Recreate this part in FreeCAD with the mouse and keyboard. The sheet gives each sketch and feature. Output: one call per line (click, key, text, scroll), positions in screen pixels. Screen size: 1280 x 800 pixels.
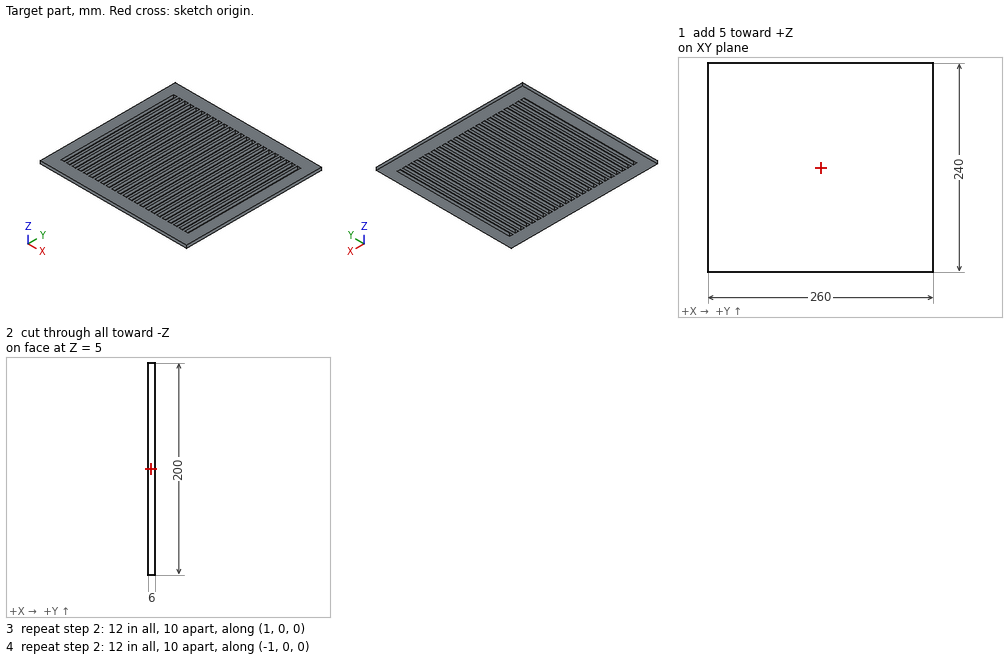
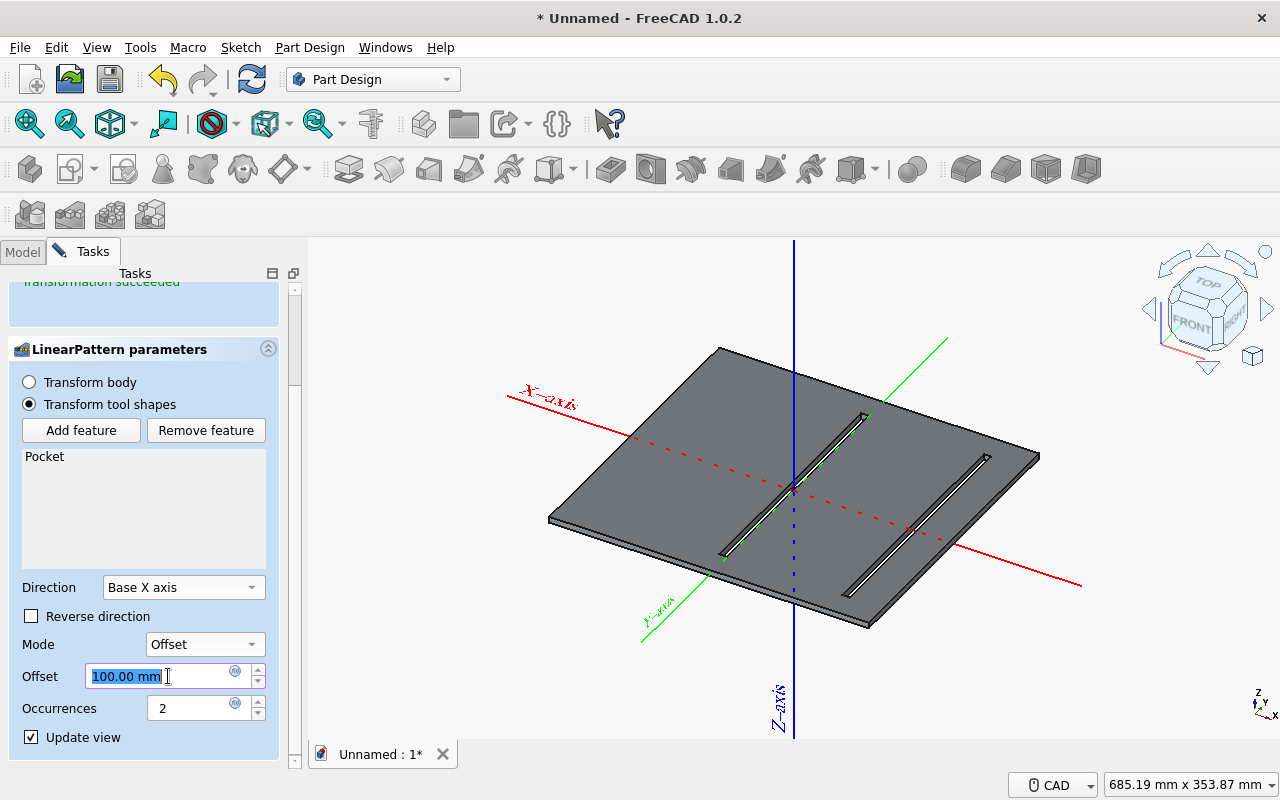
text(10)
key(Tab)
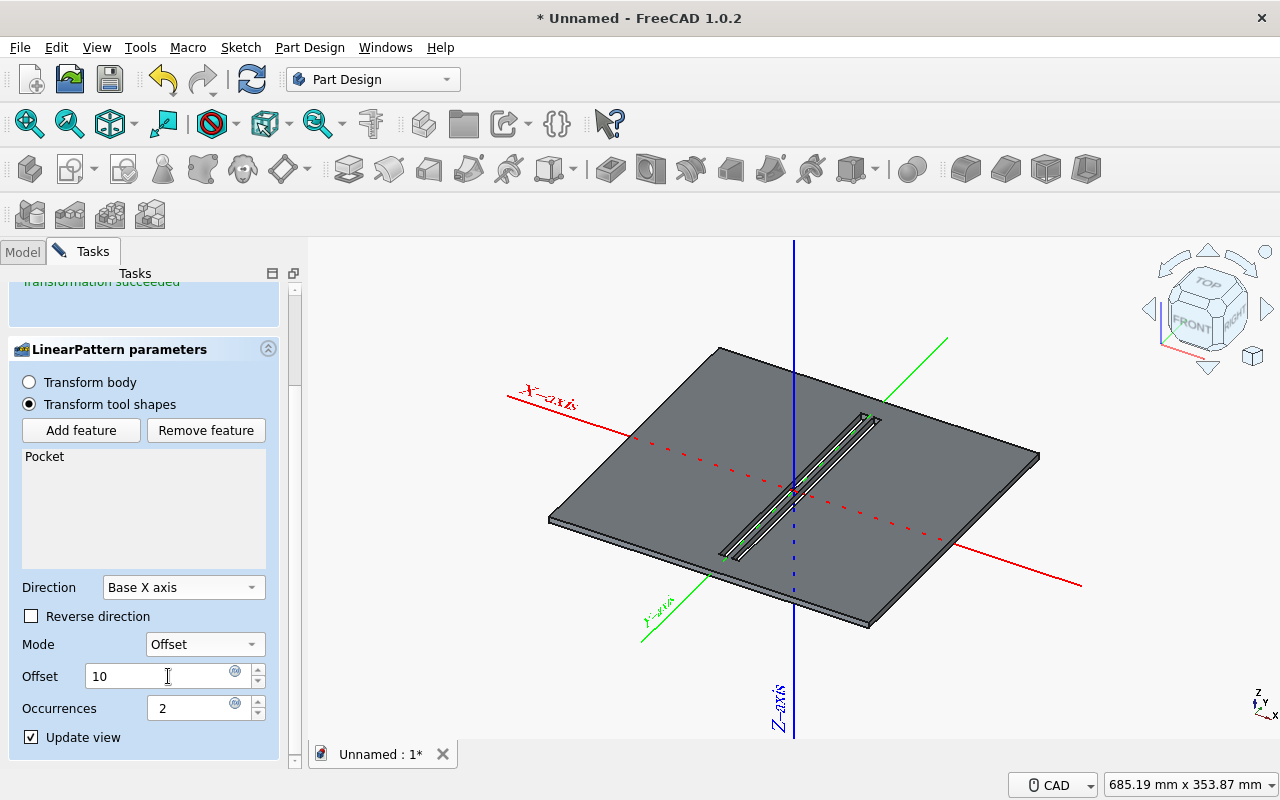
triple_click(198, 708)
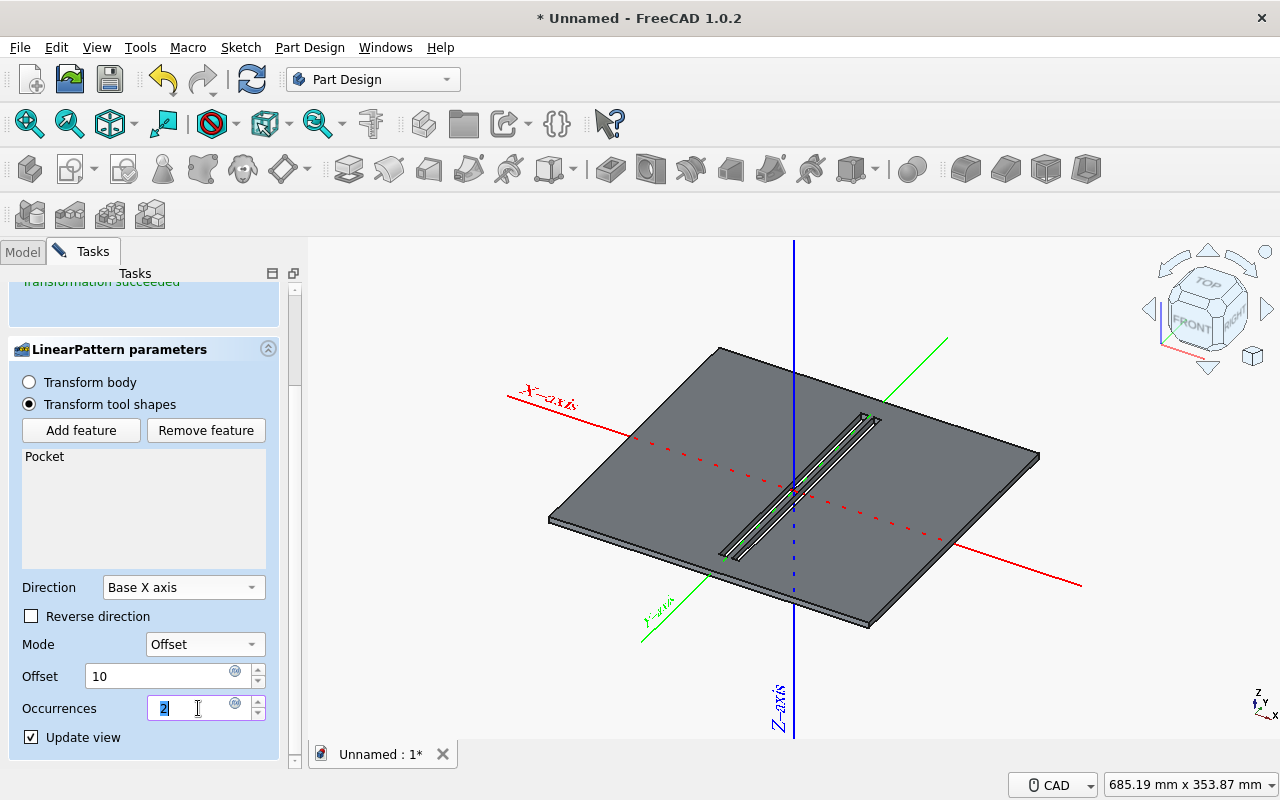
text(12)
key(Tab)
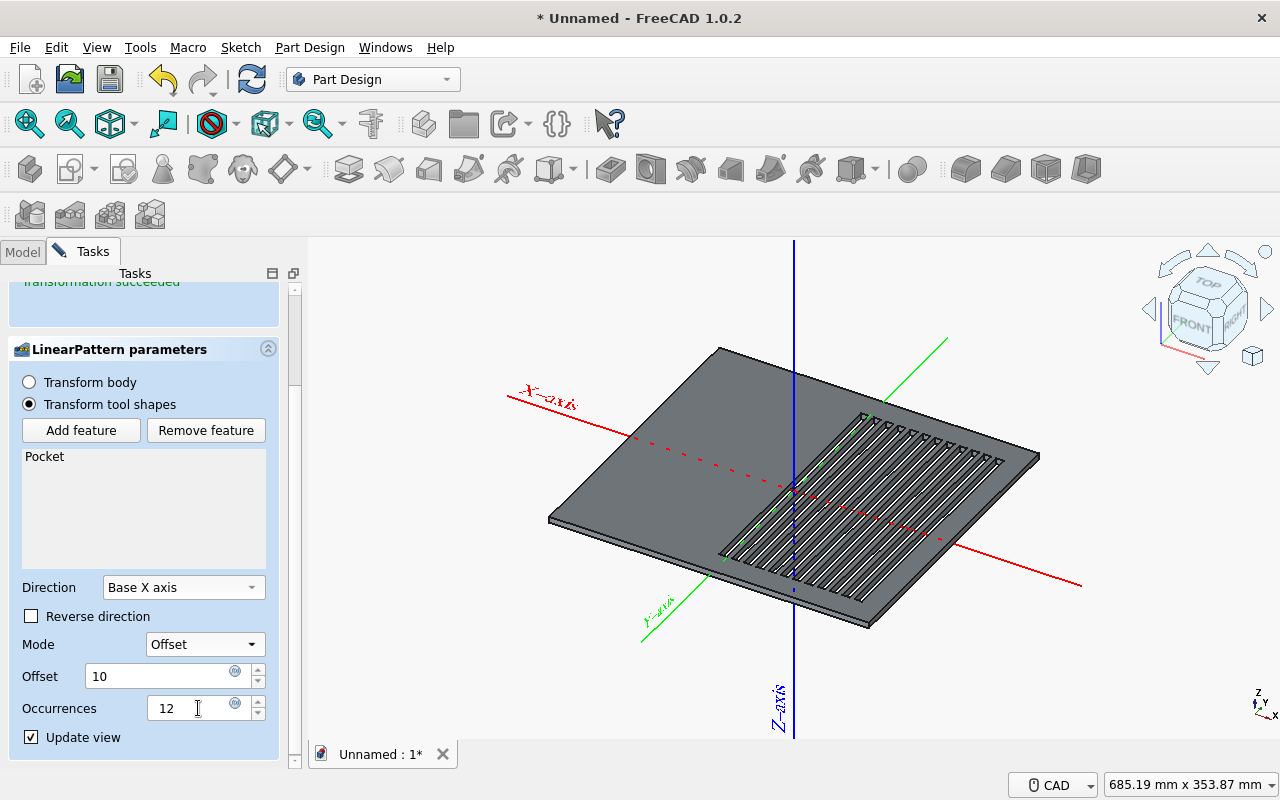
scroll(295, 526, up, 3)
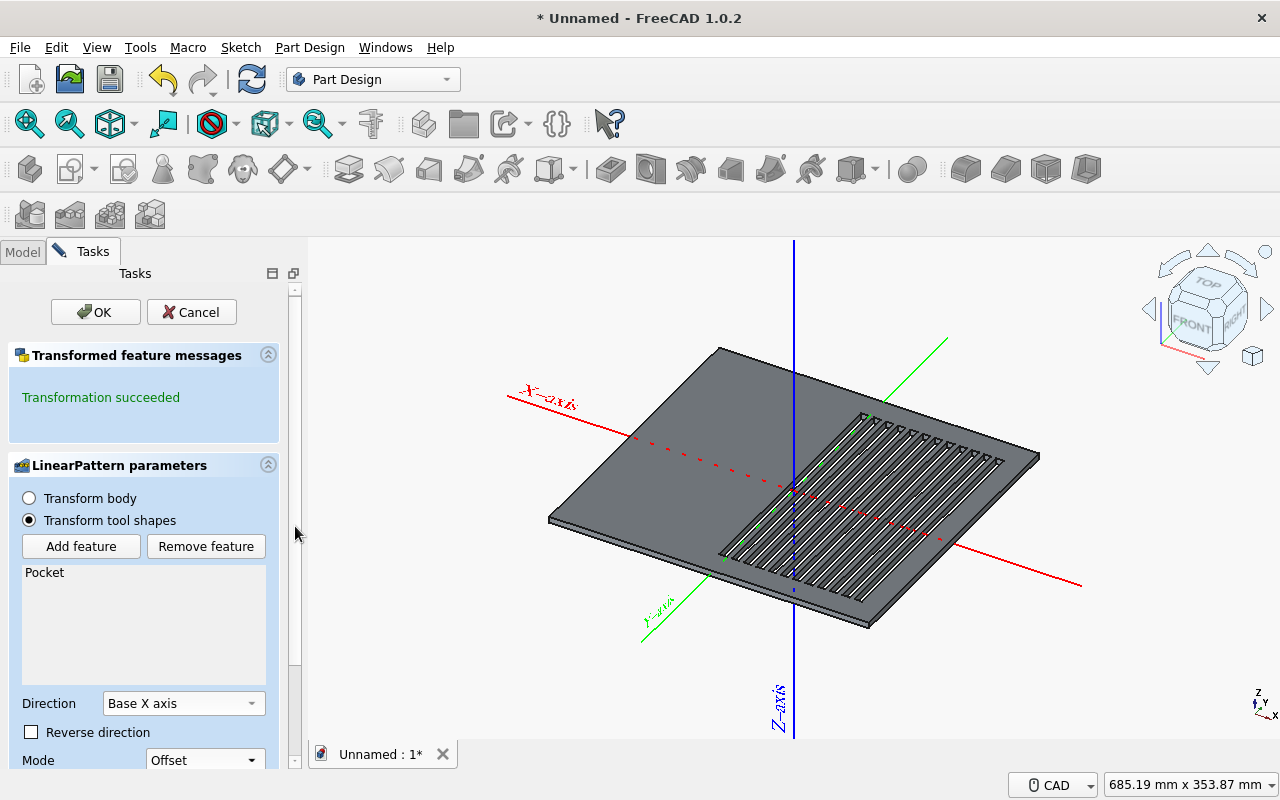
click(96, 312)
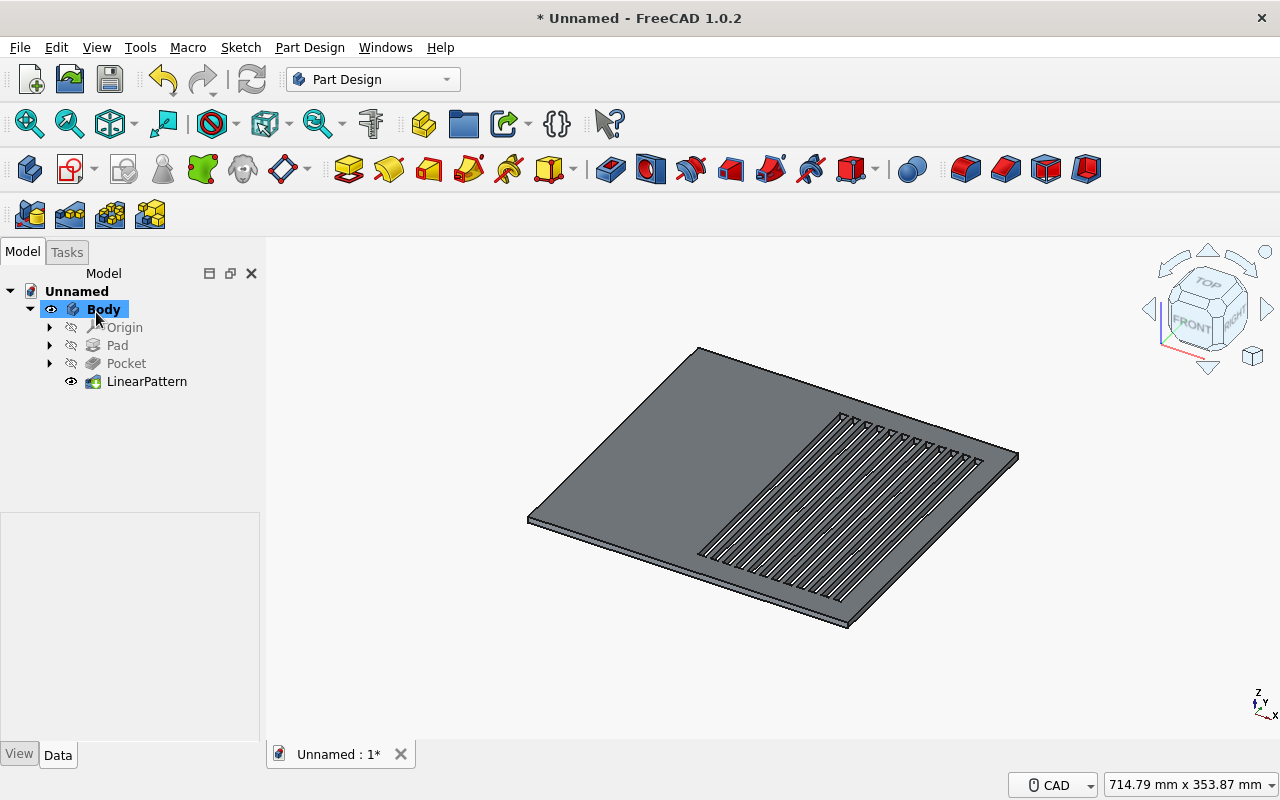
click(116, 363)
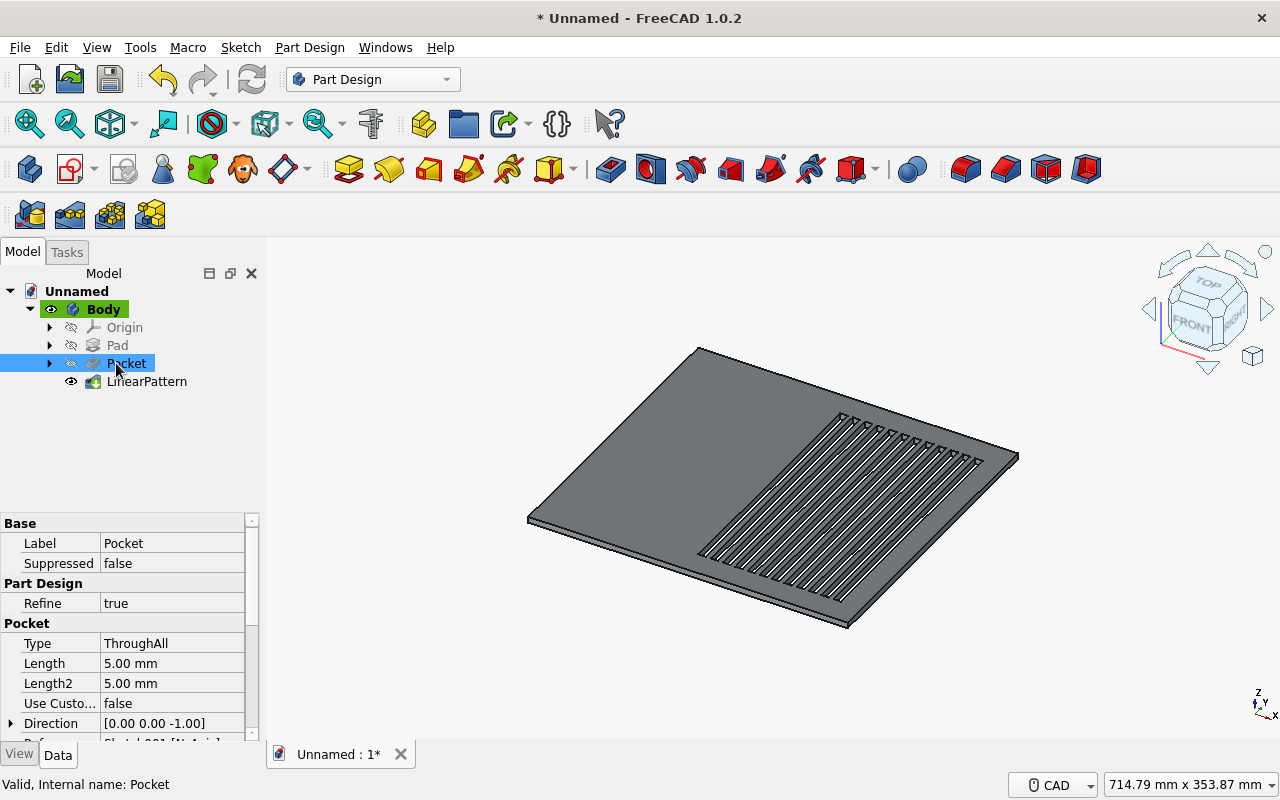
click(70, 214)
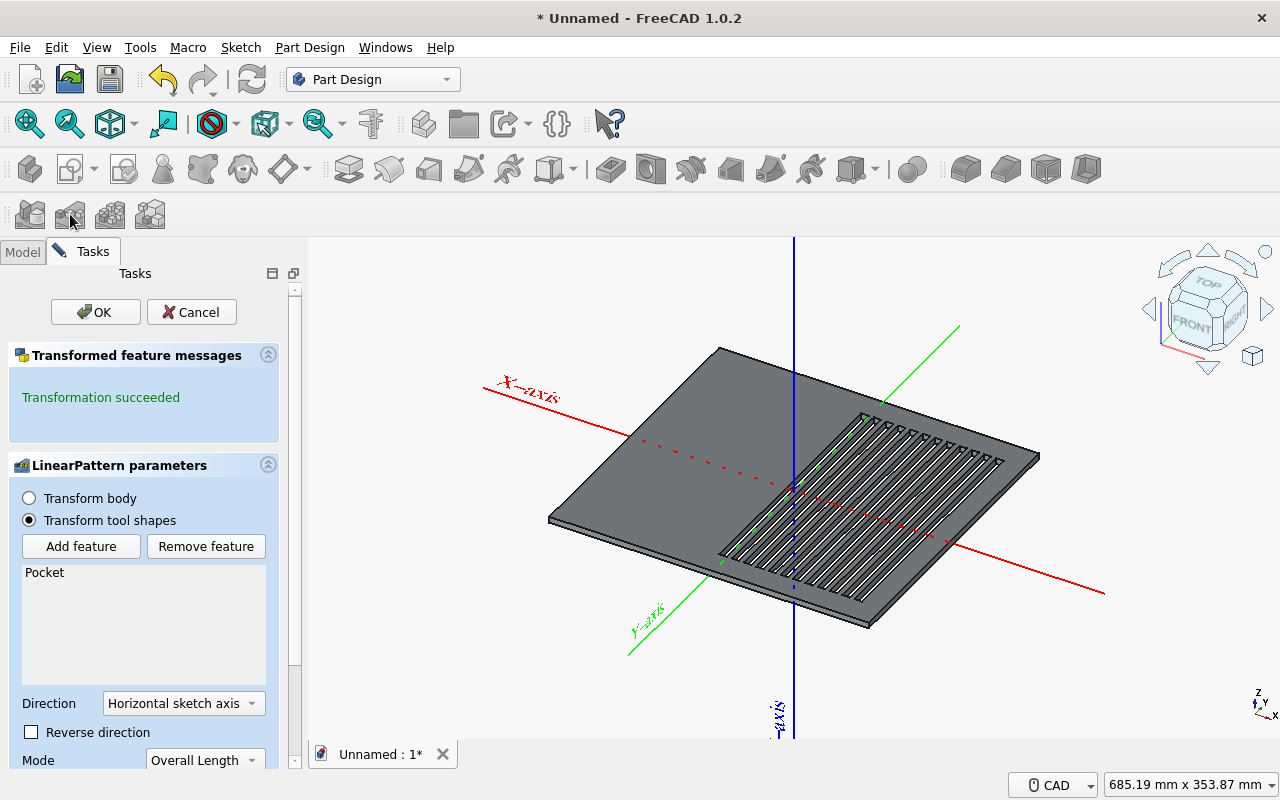
click(184, 704)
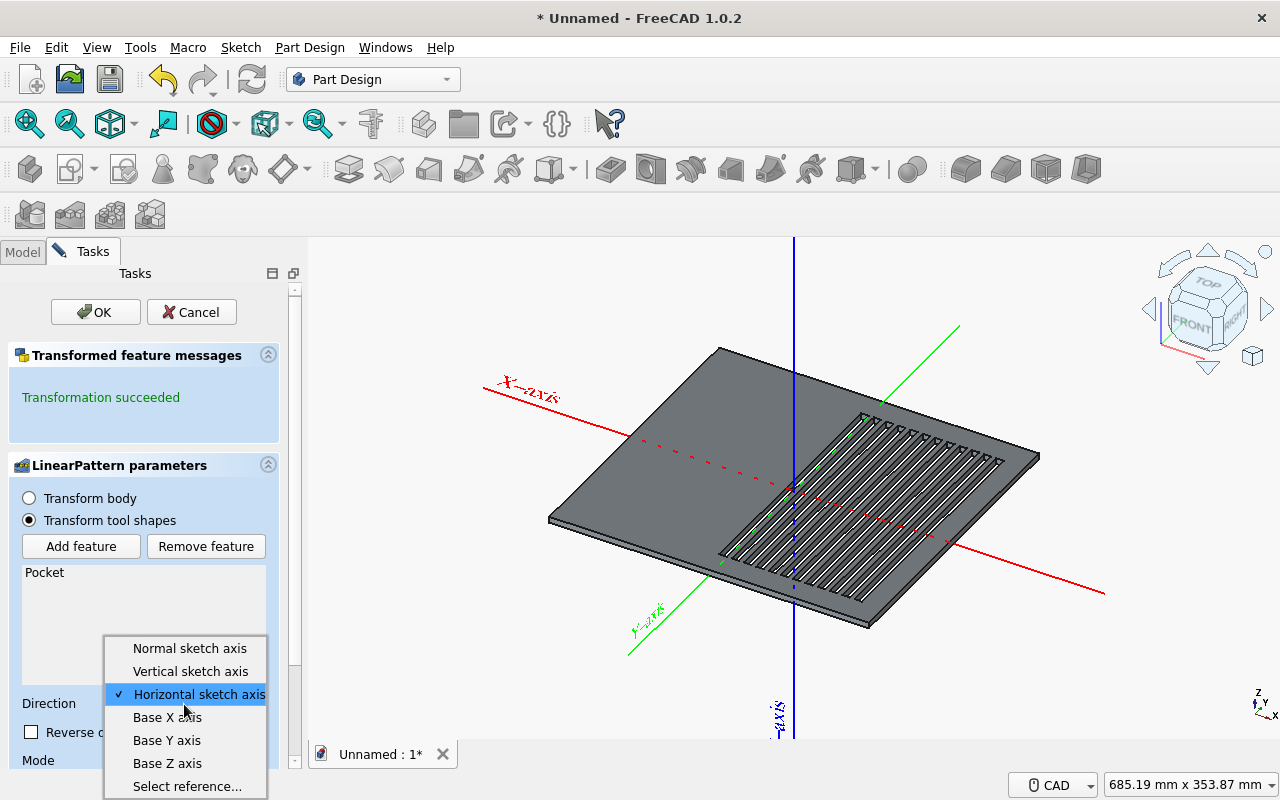
click(184, 718)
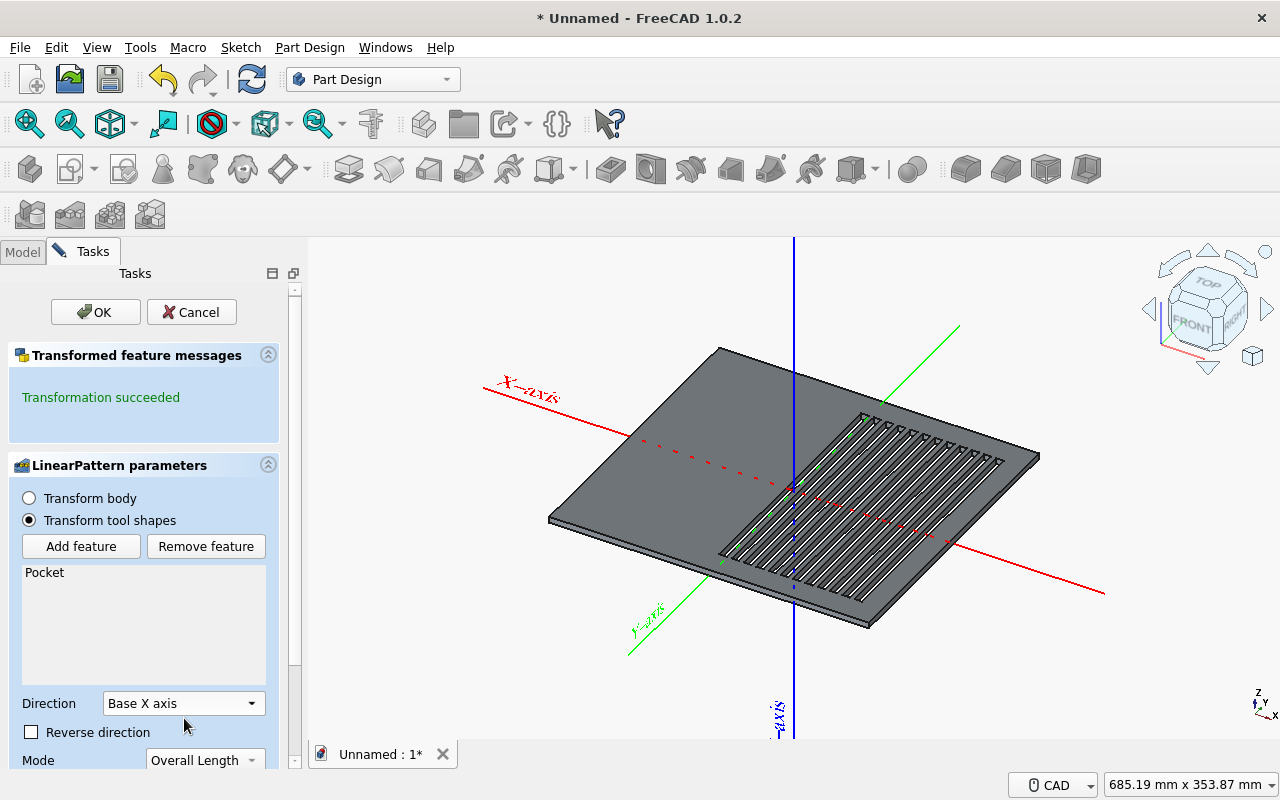
scroll(295, 526, down, 2)